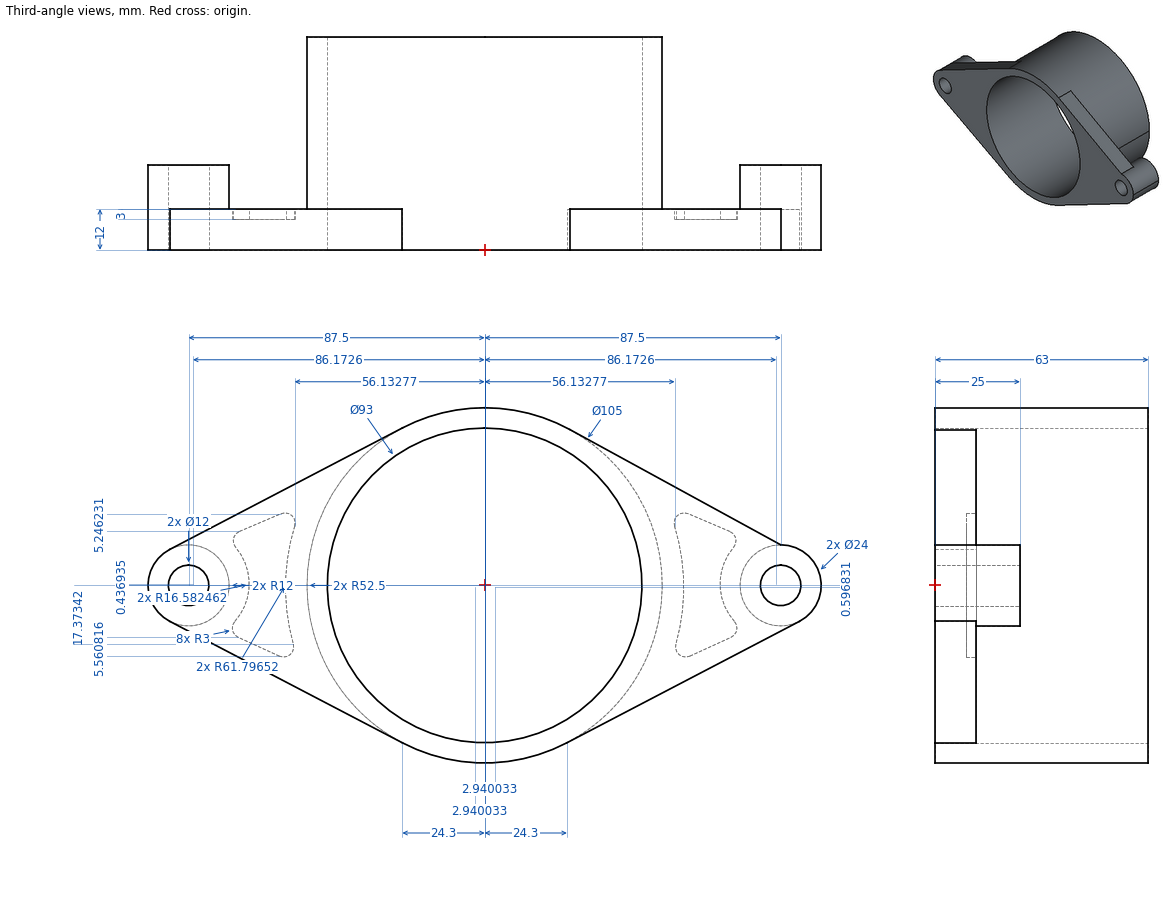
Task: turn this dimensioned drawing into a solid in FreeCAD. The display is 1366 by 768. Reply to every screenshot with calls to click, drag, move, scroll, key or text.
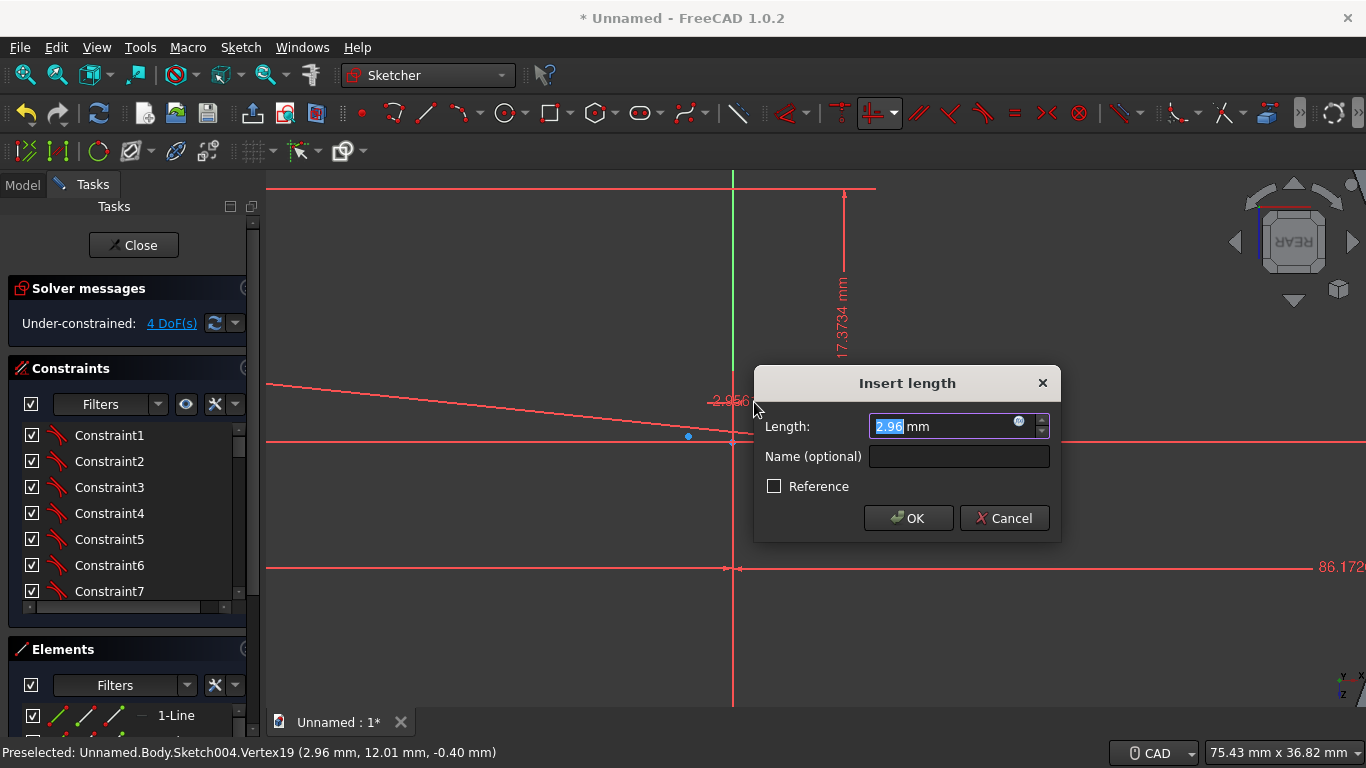
text(2.940033)
key(Return)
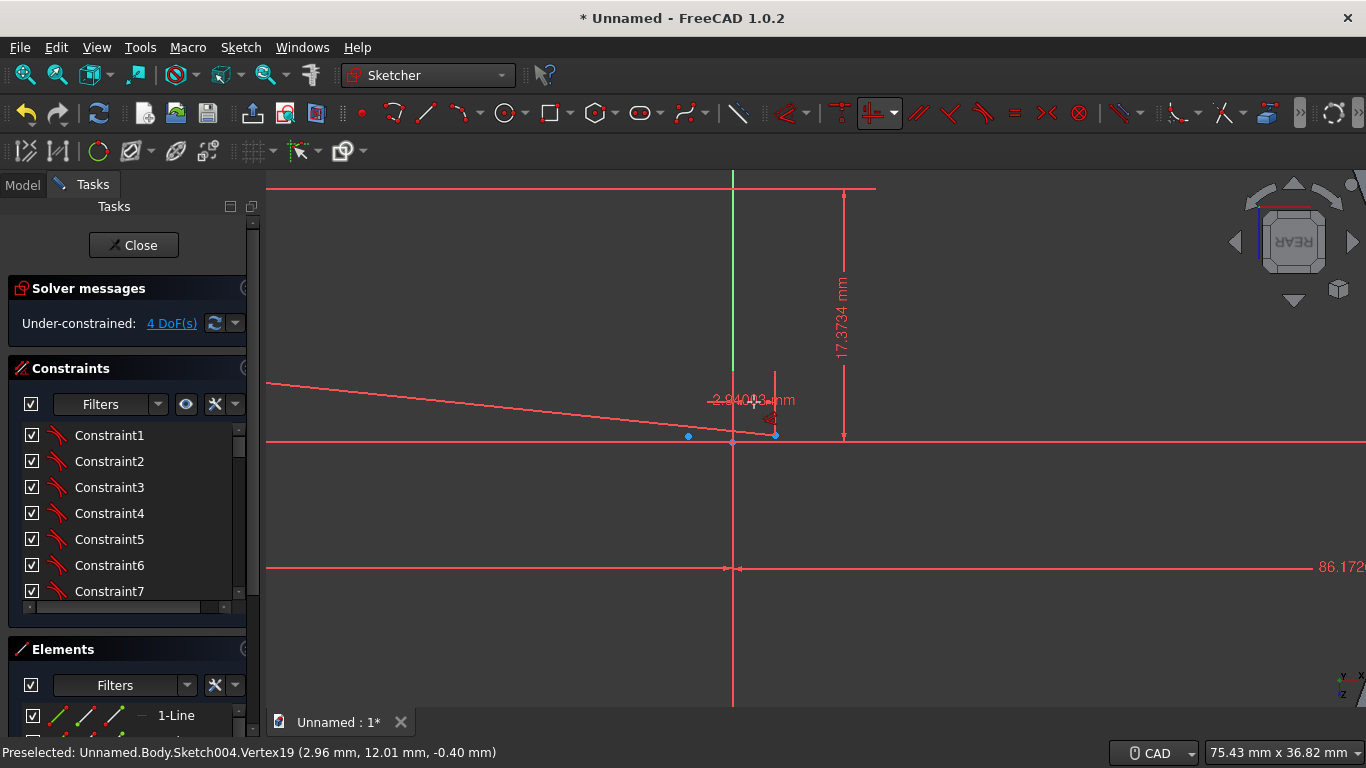
scroll(775, 436, up, 8)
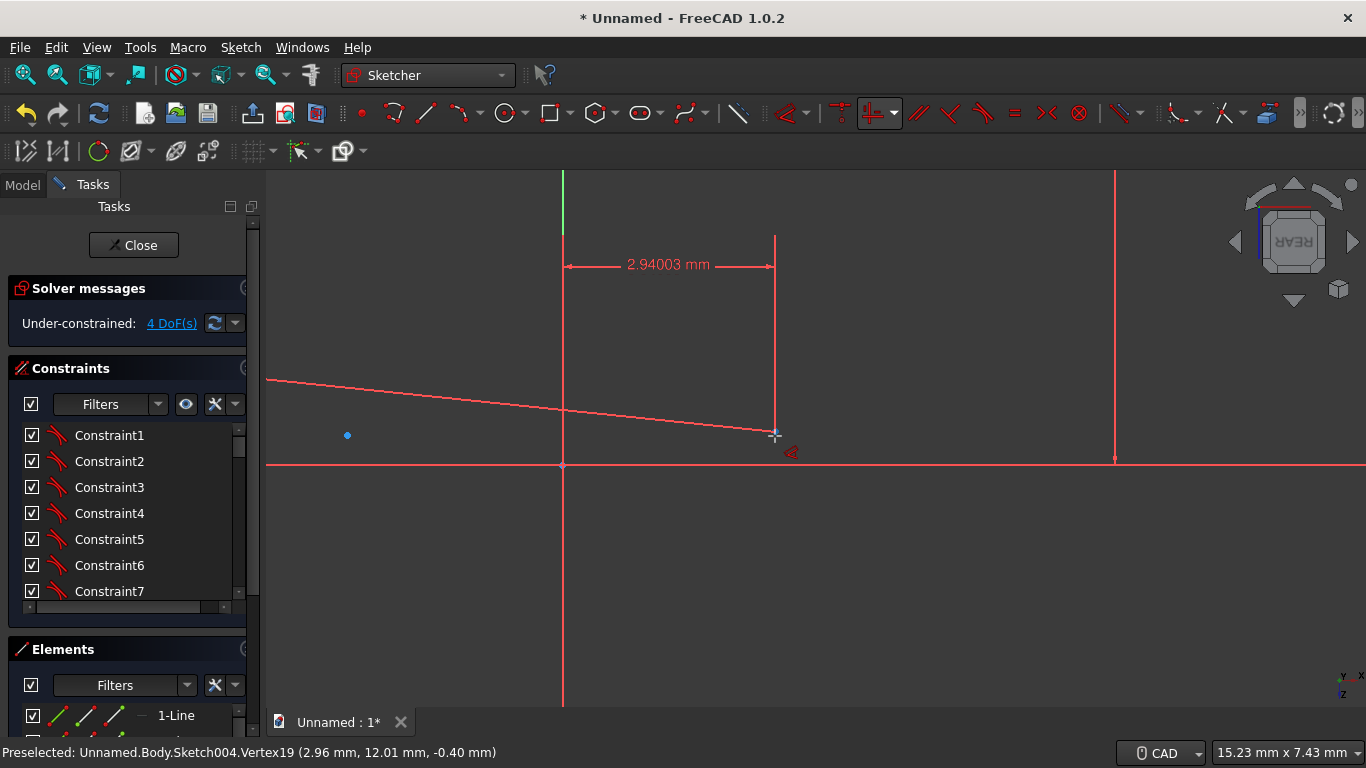
click(775, 432)
click(809, 448)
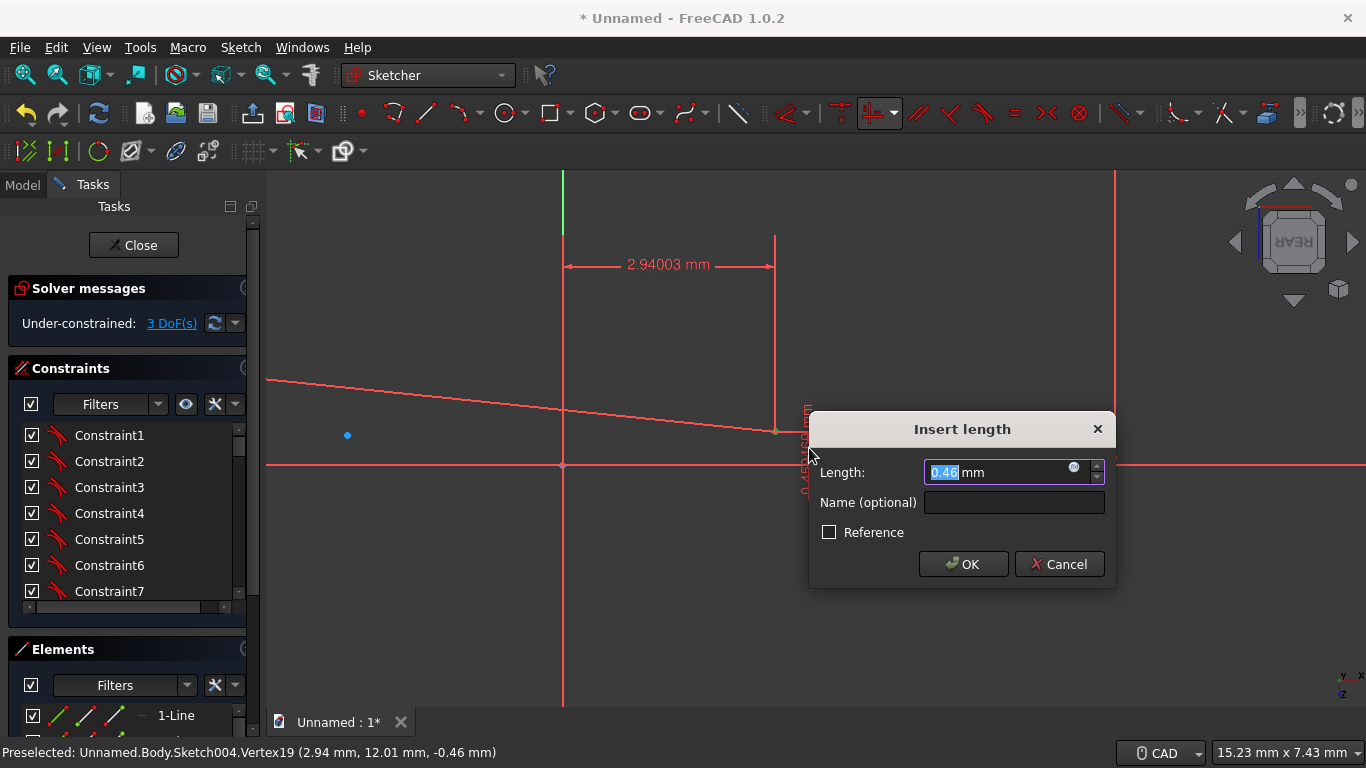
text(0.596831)
key(Return)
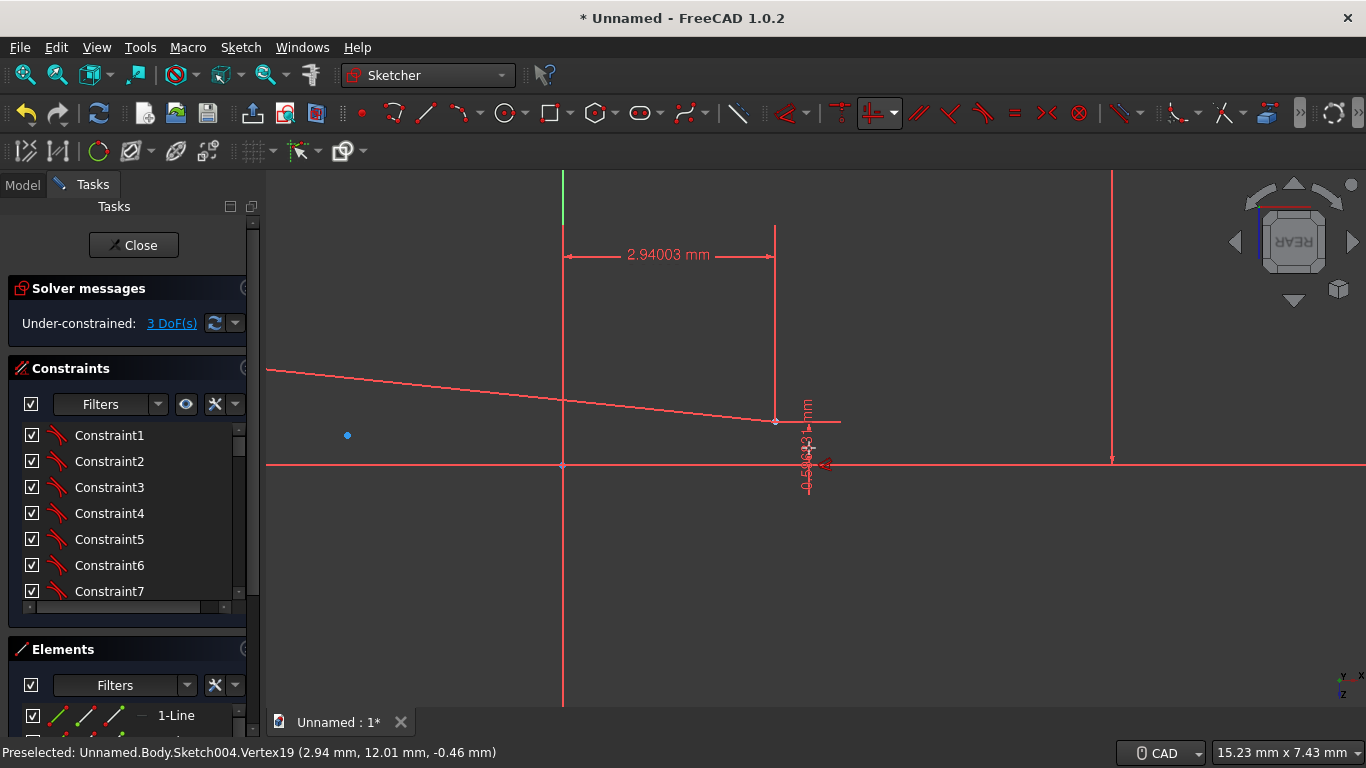
scroll(759, 436, down, 14)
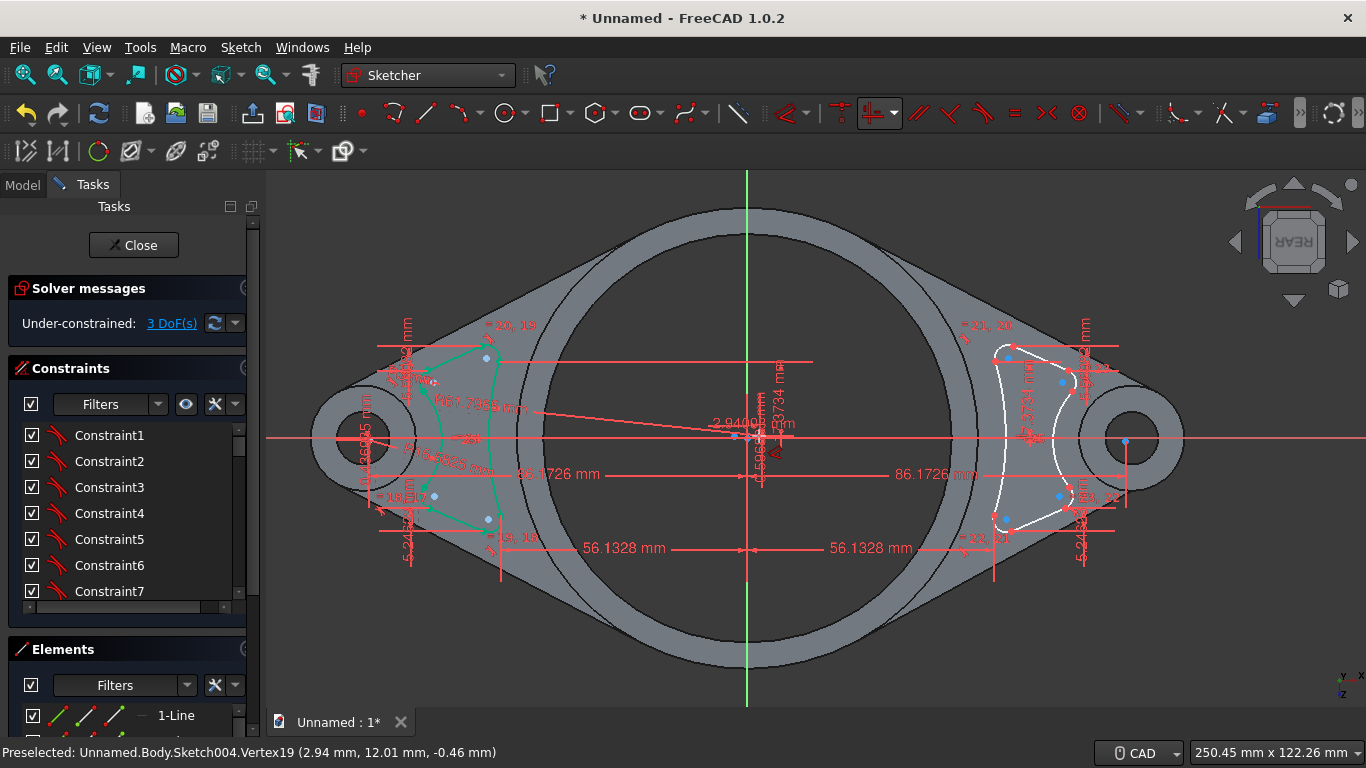
scroll(734, 436, up, 6)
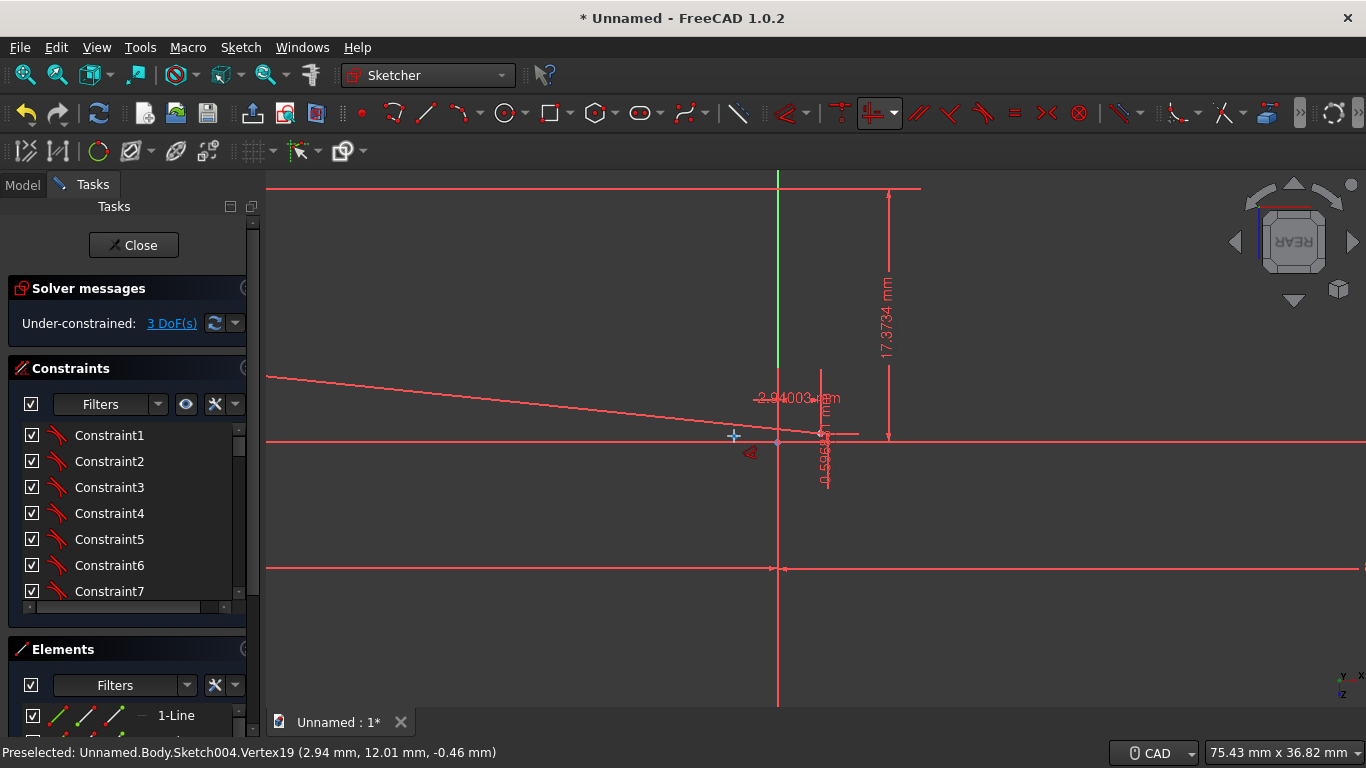
click(734, 436)
click(756, 476)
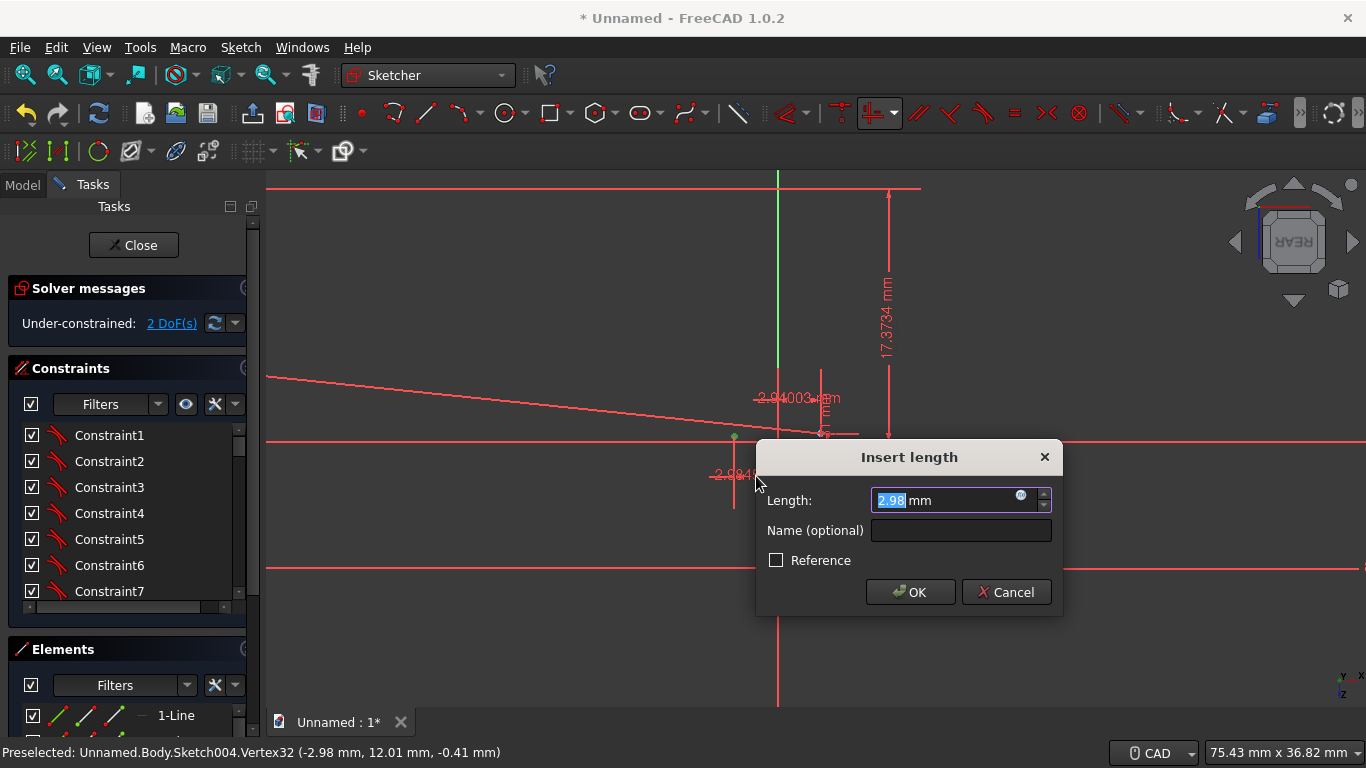
text(2.940033)
key(Return)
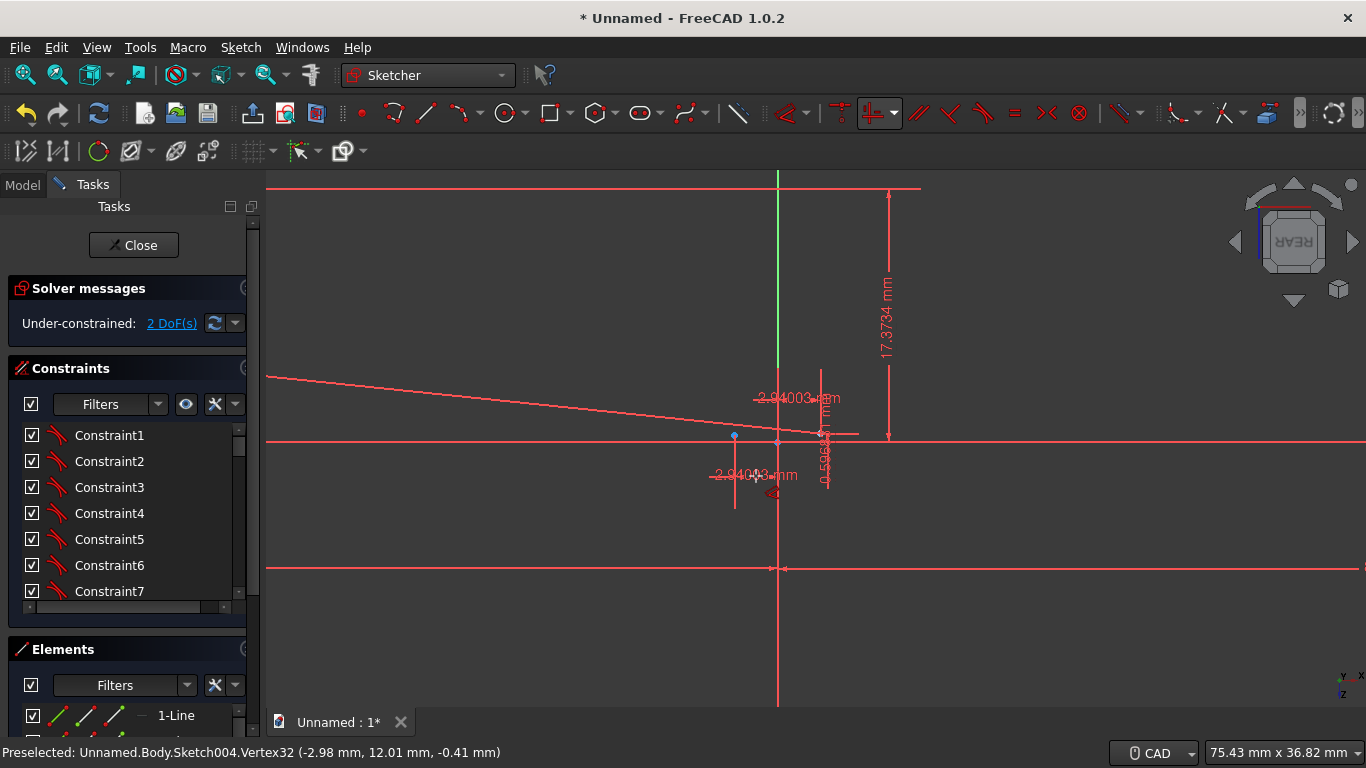
scroll(735, 435, up, 8)